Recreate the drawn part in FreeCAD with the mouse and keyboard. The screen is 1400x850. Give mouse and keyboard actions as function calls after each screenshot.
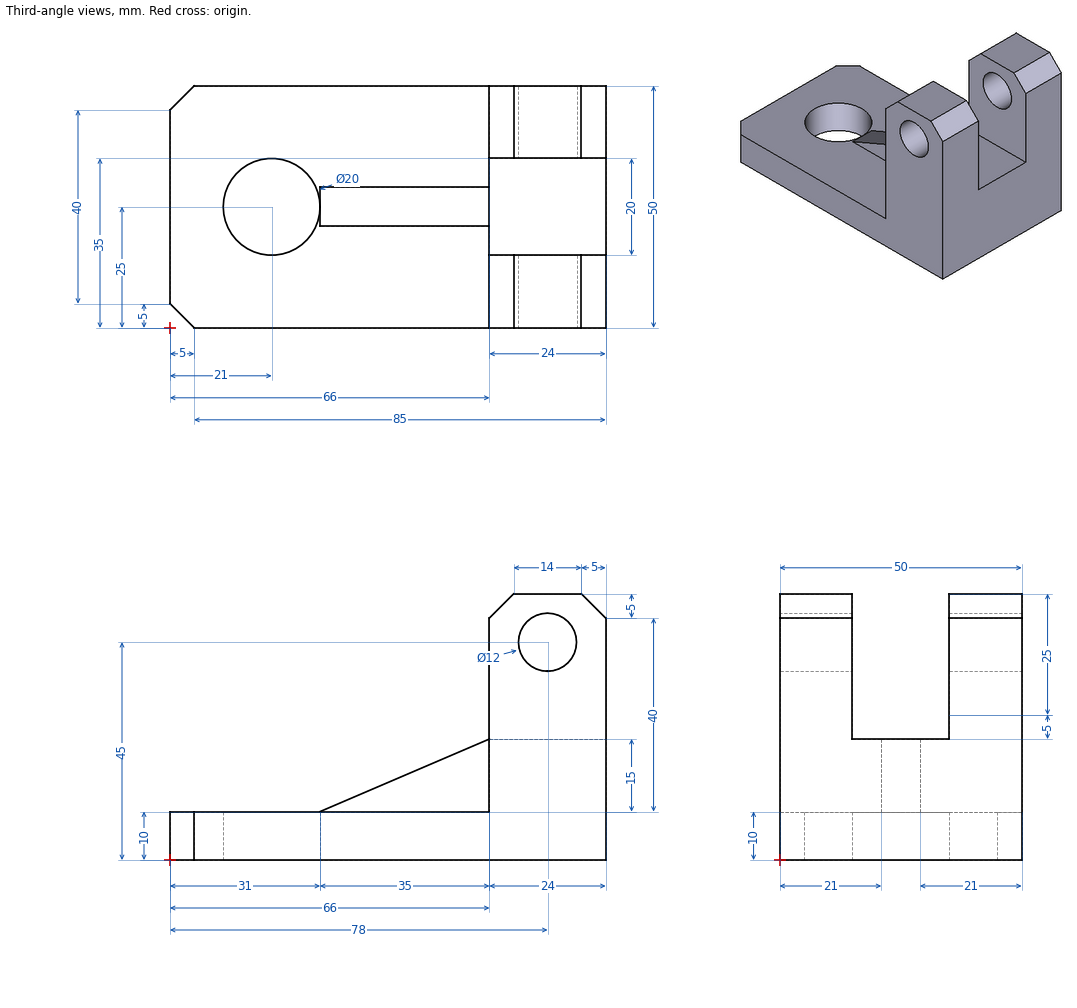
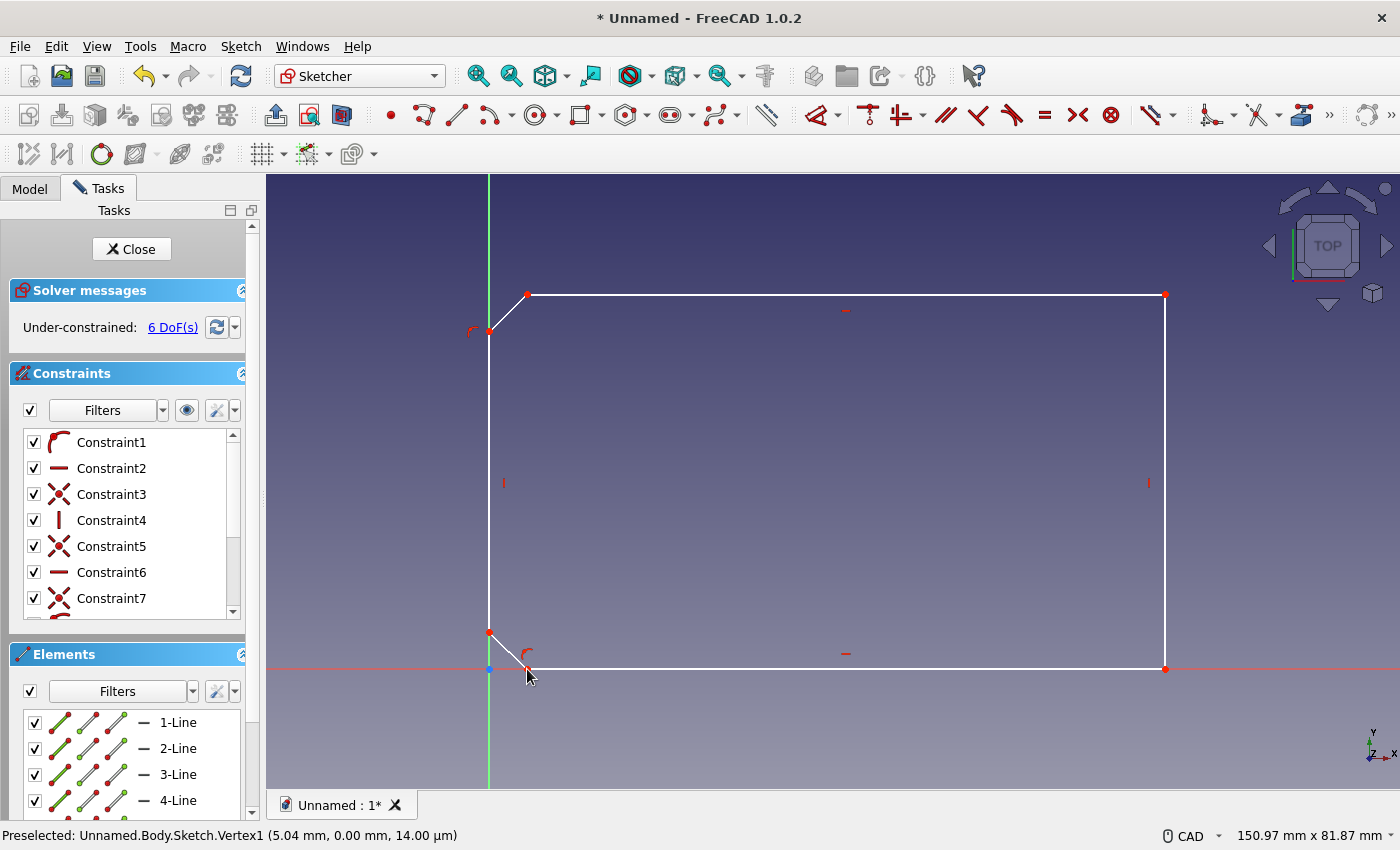
click(816, 116)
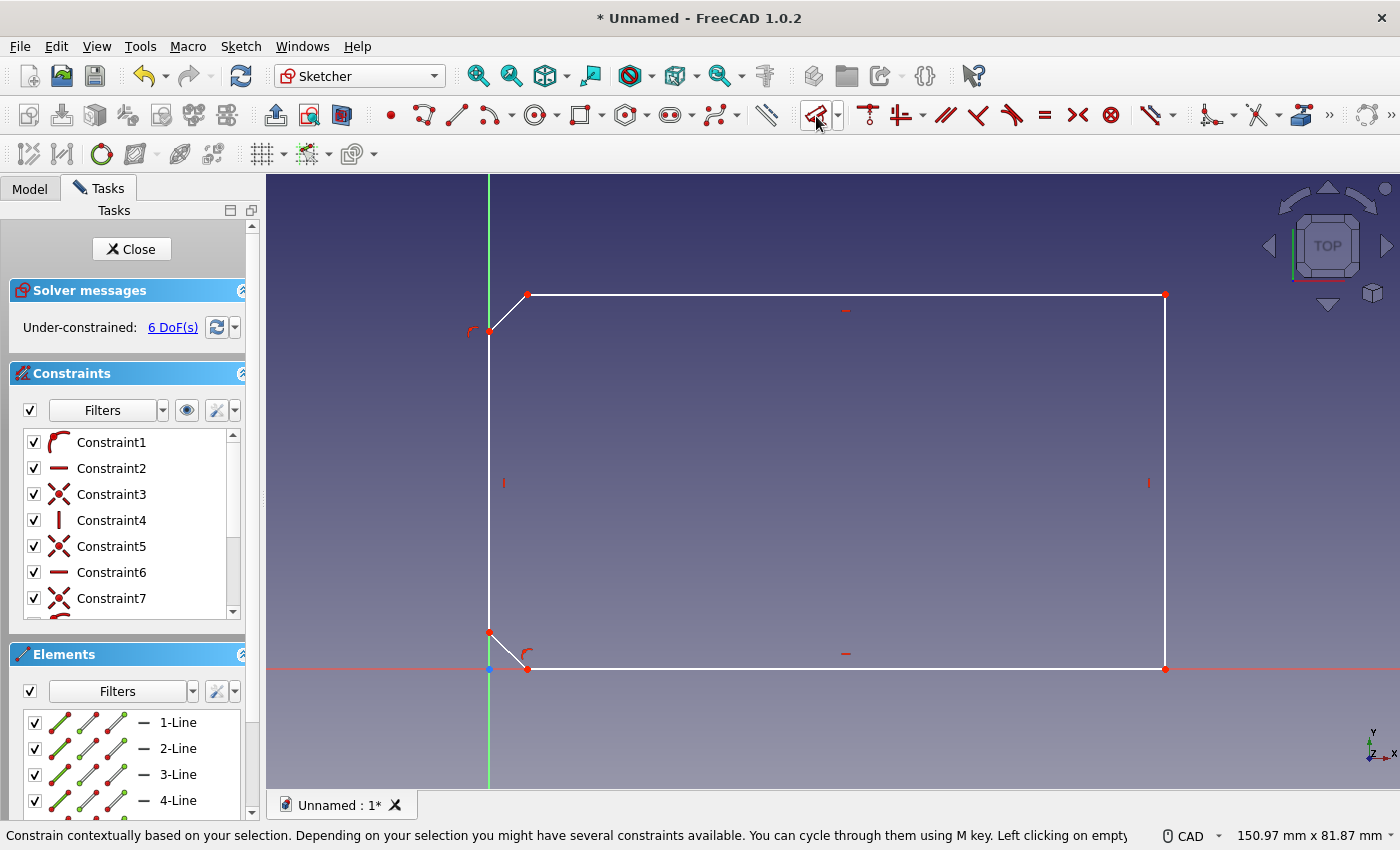
click(718, 669)
click(846, 703)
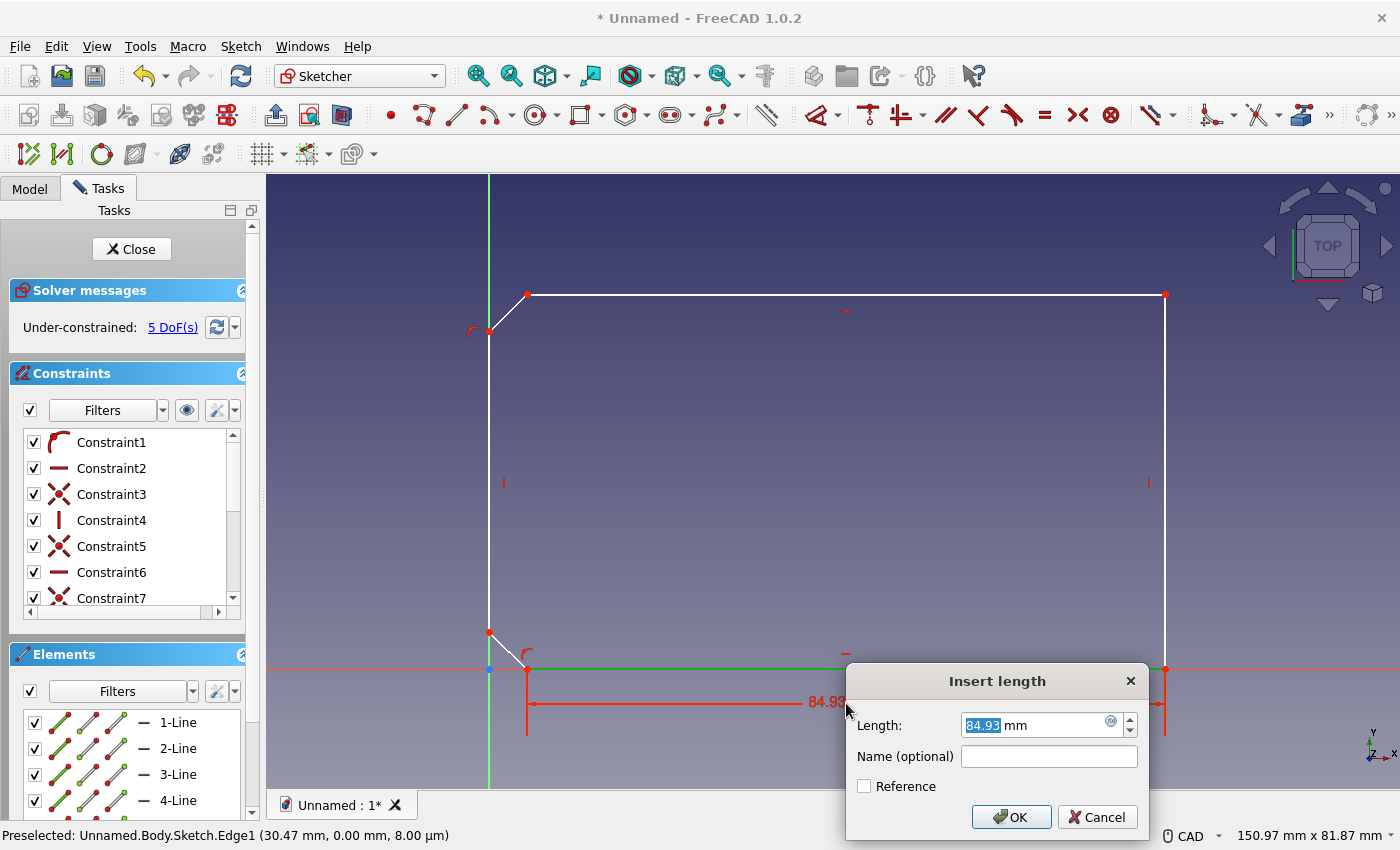
text(85)
key(Return)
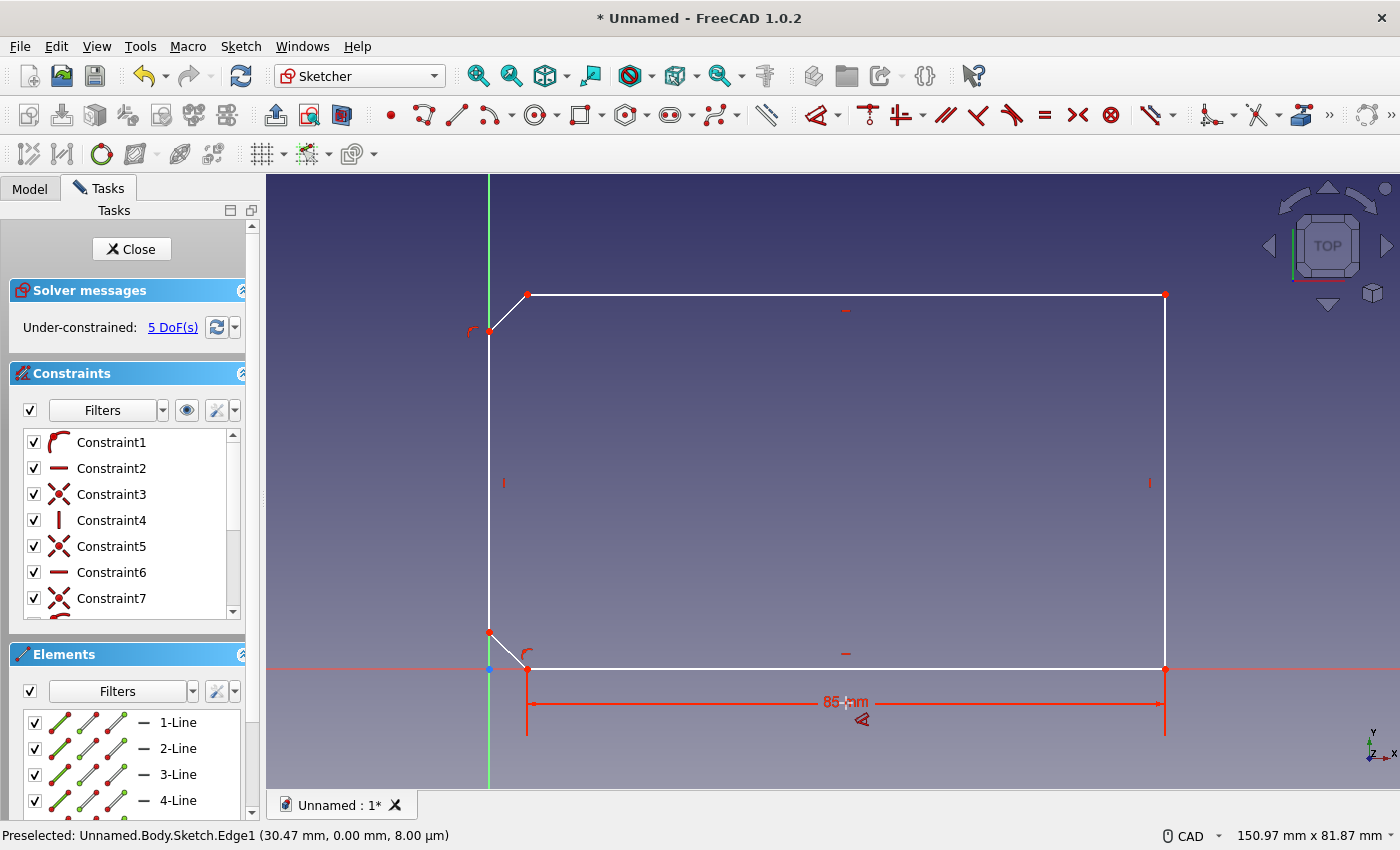
click(1165, 557)
click(1199, 482)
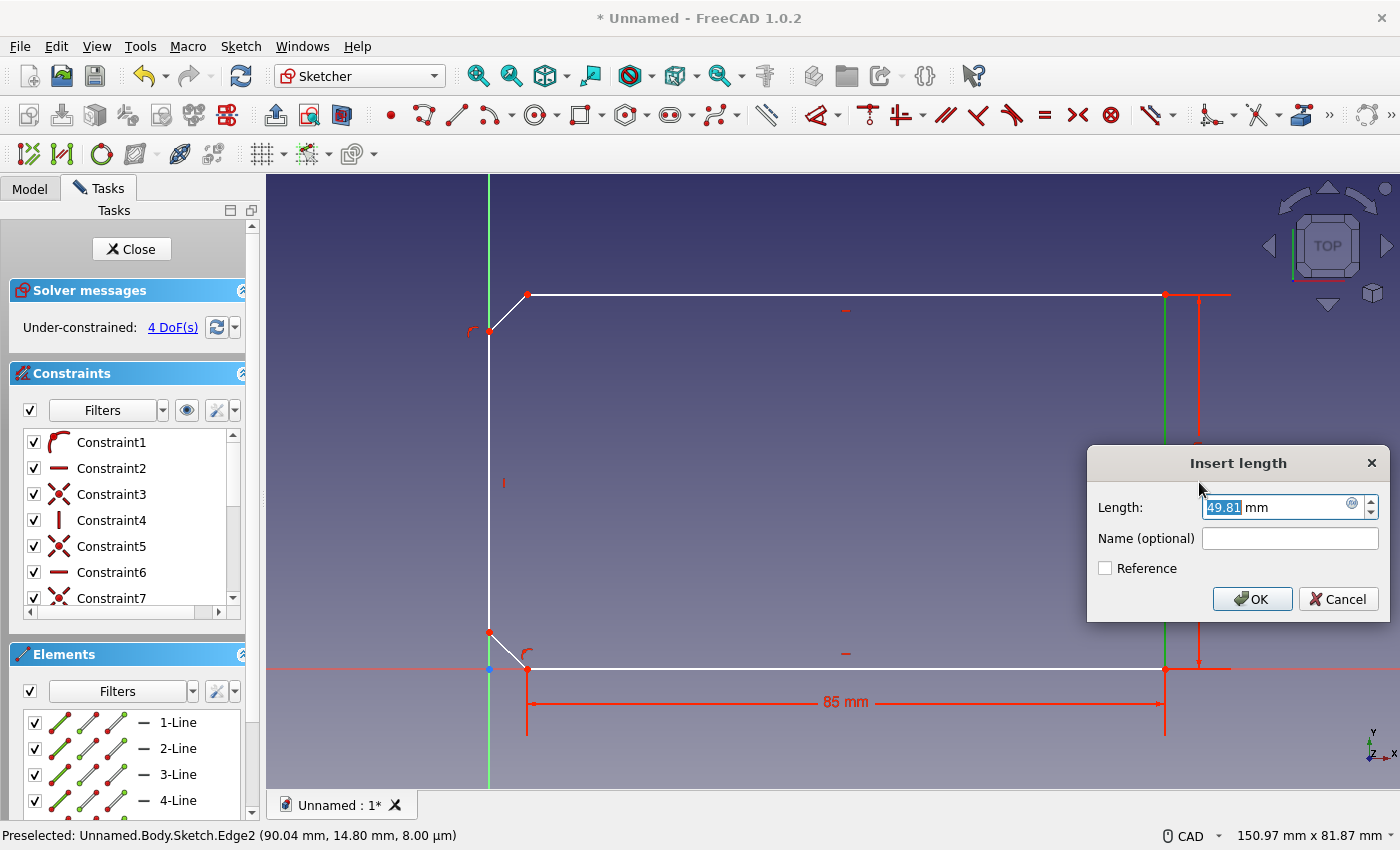
text(50)
key(Return)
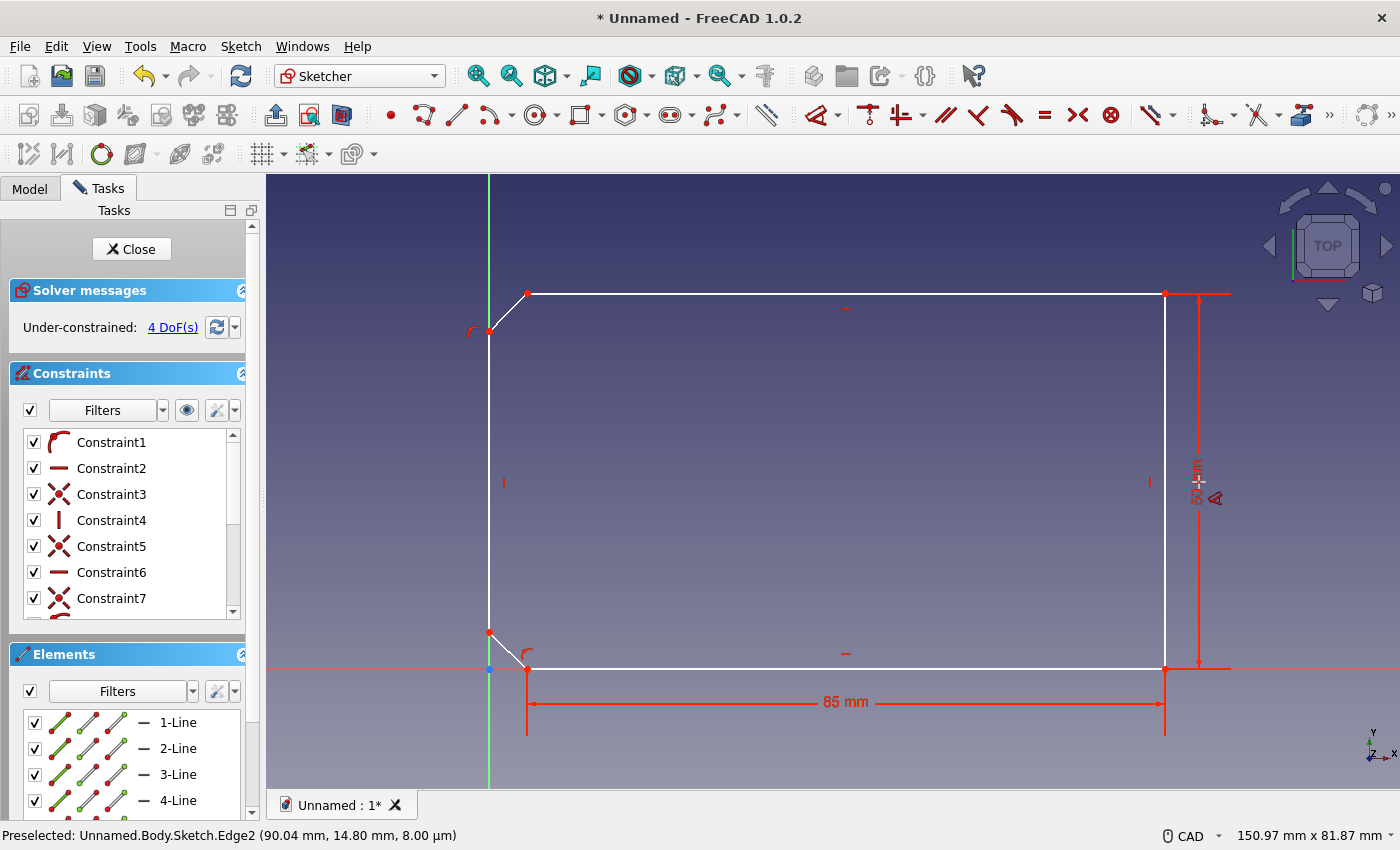
click(974, 294)
click(846, 260)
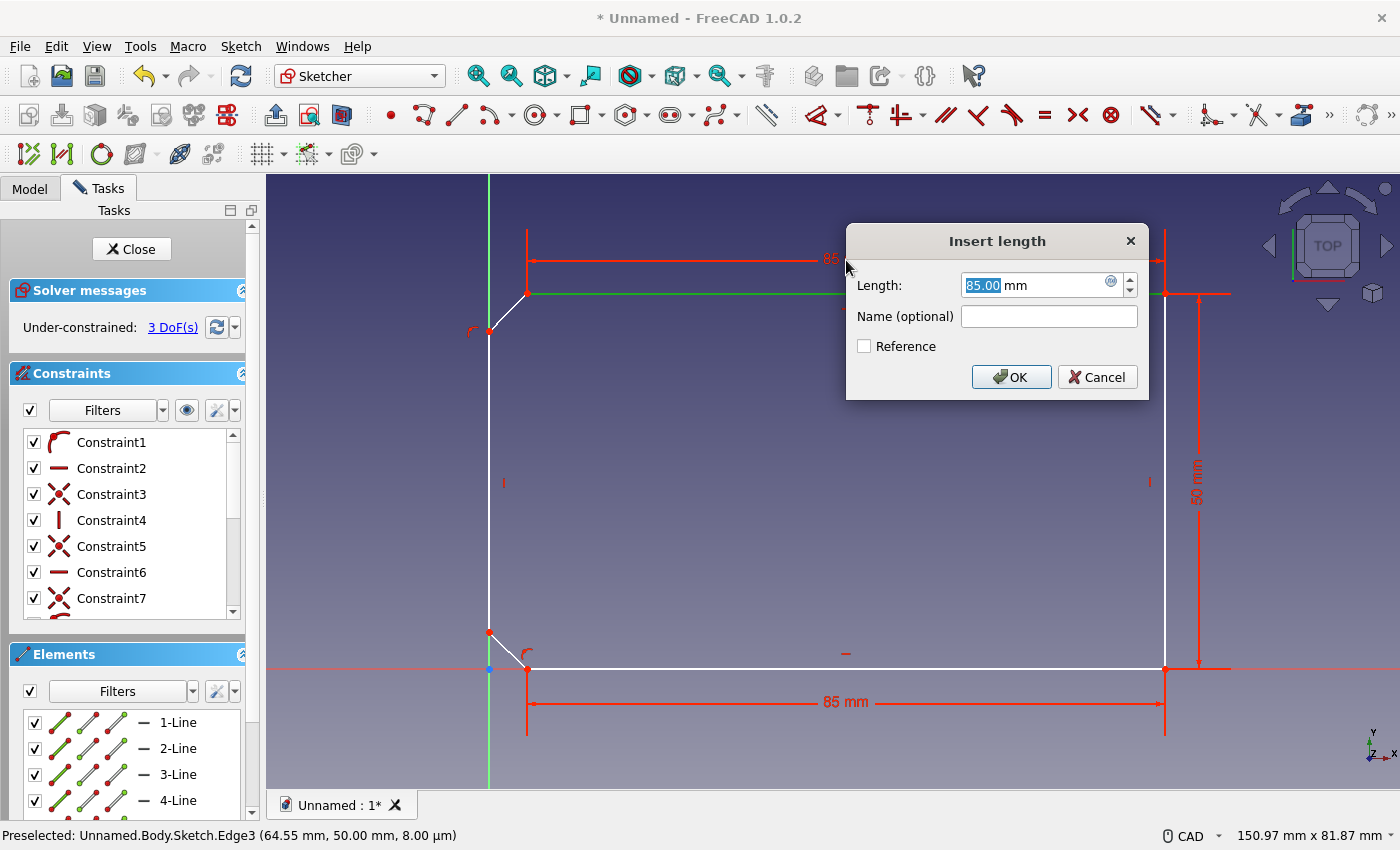
text(85)
key(Return)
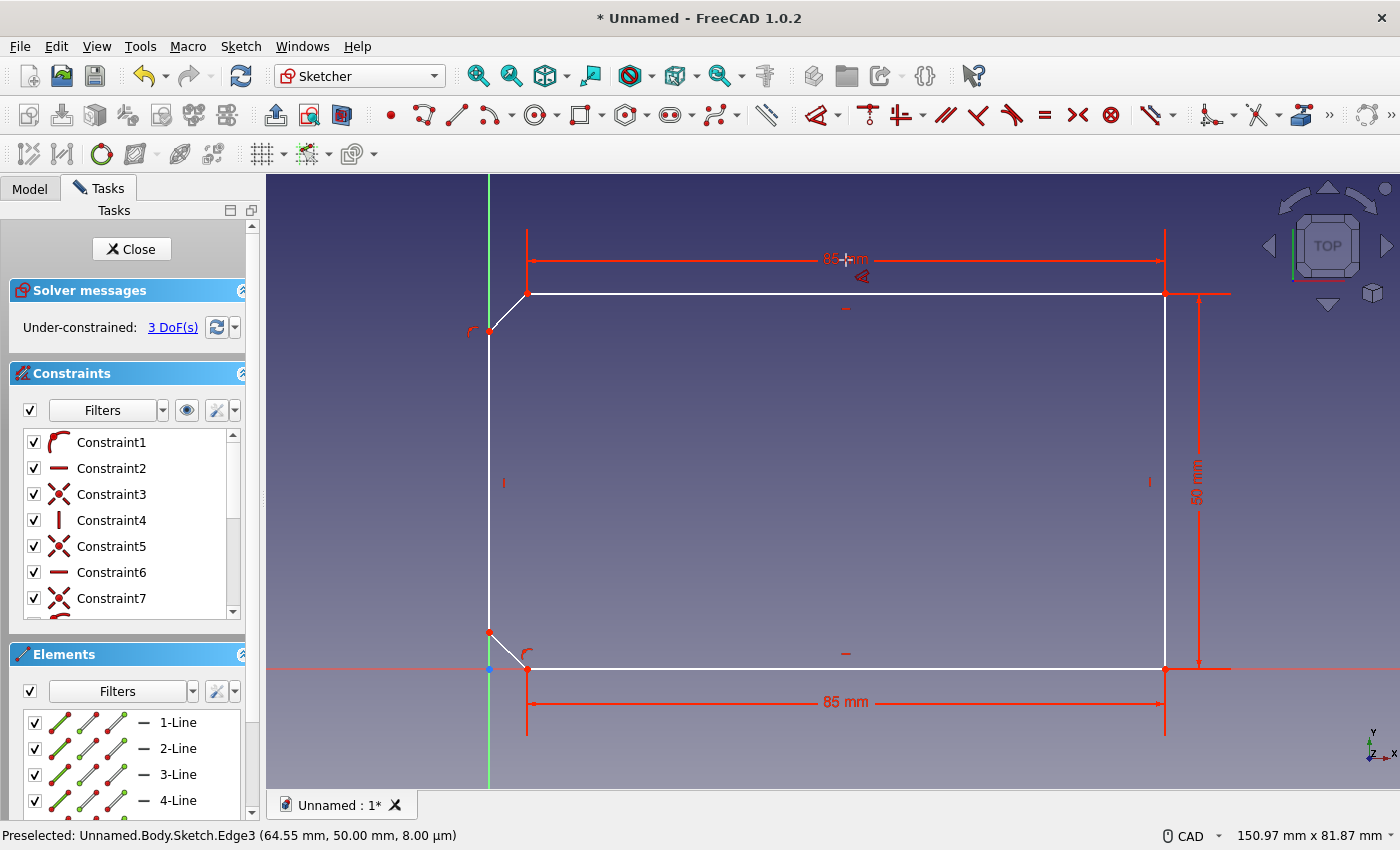
click(489, 422)
click(455, 482)